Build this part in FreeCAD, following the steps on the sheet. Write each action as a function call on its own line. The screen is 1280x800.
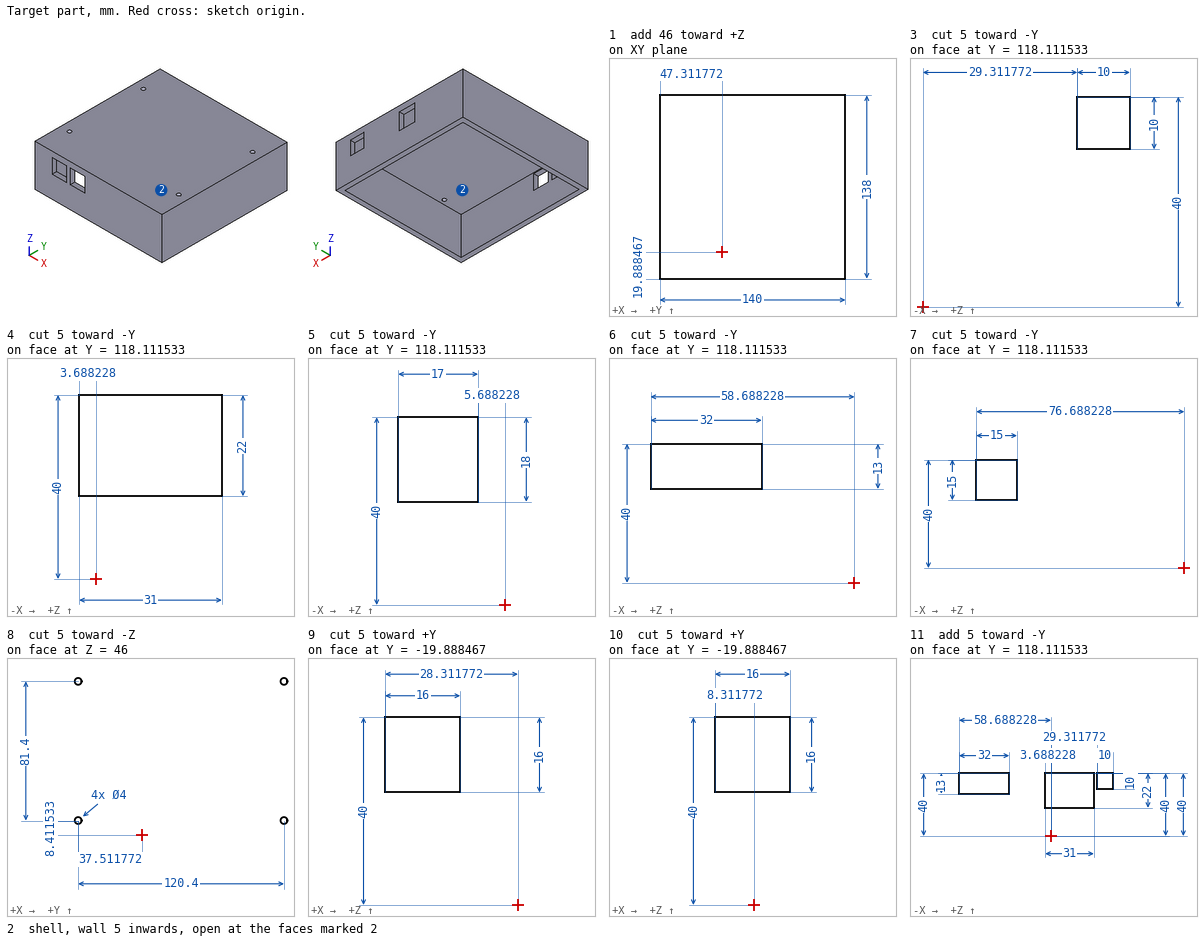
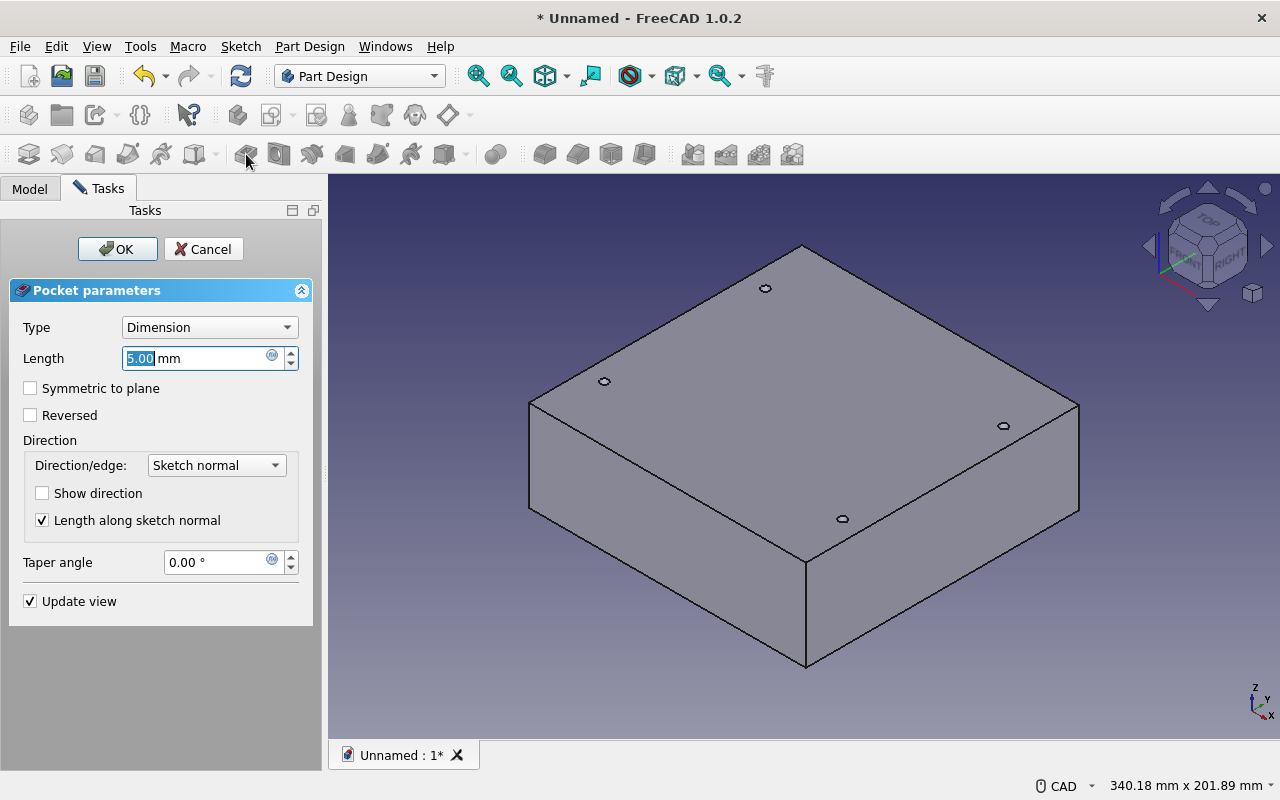
text(5)
key(Tab)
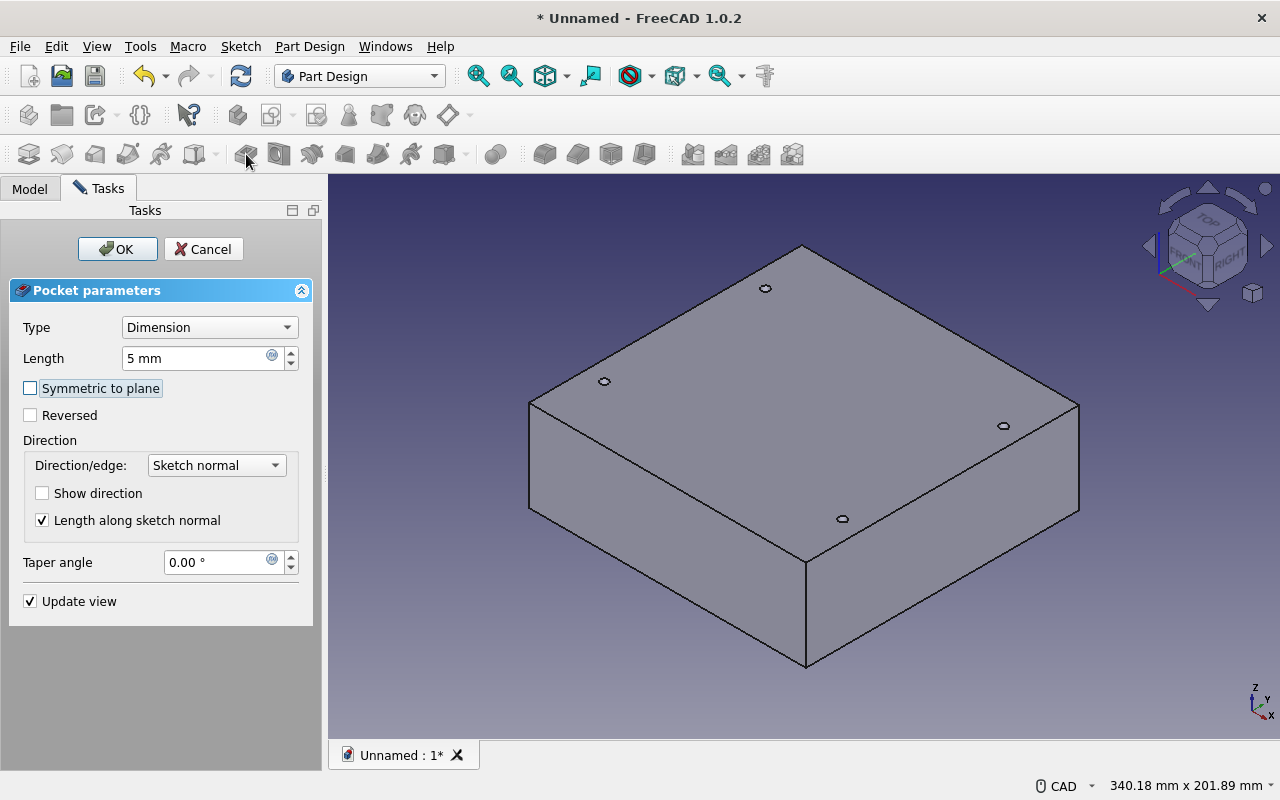
click(118, 249)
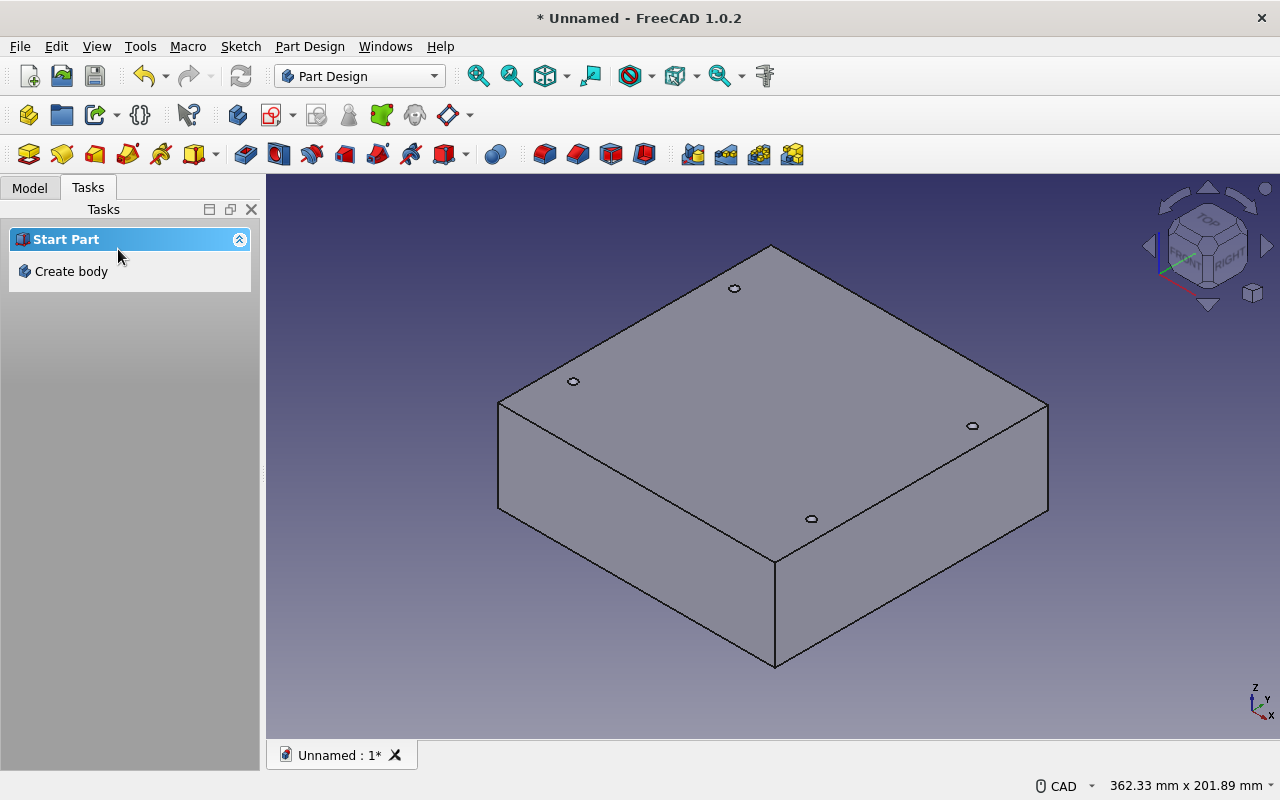
click(716, 580)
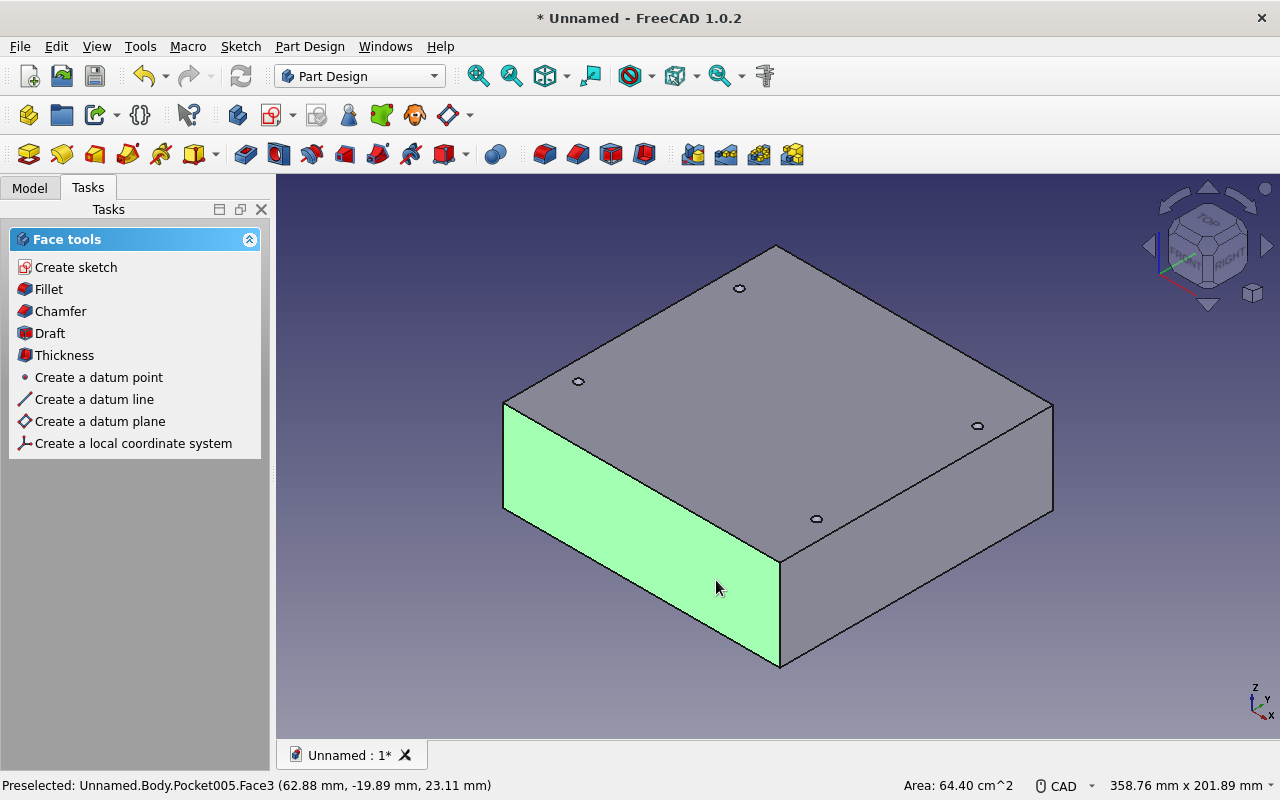
click(270, 116)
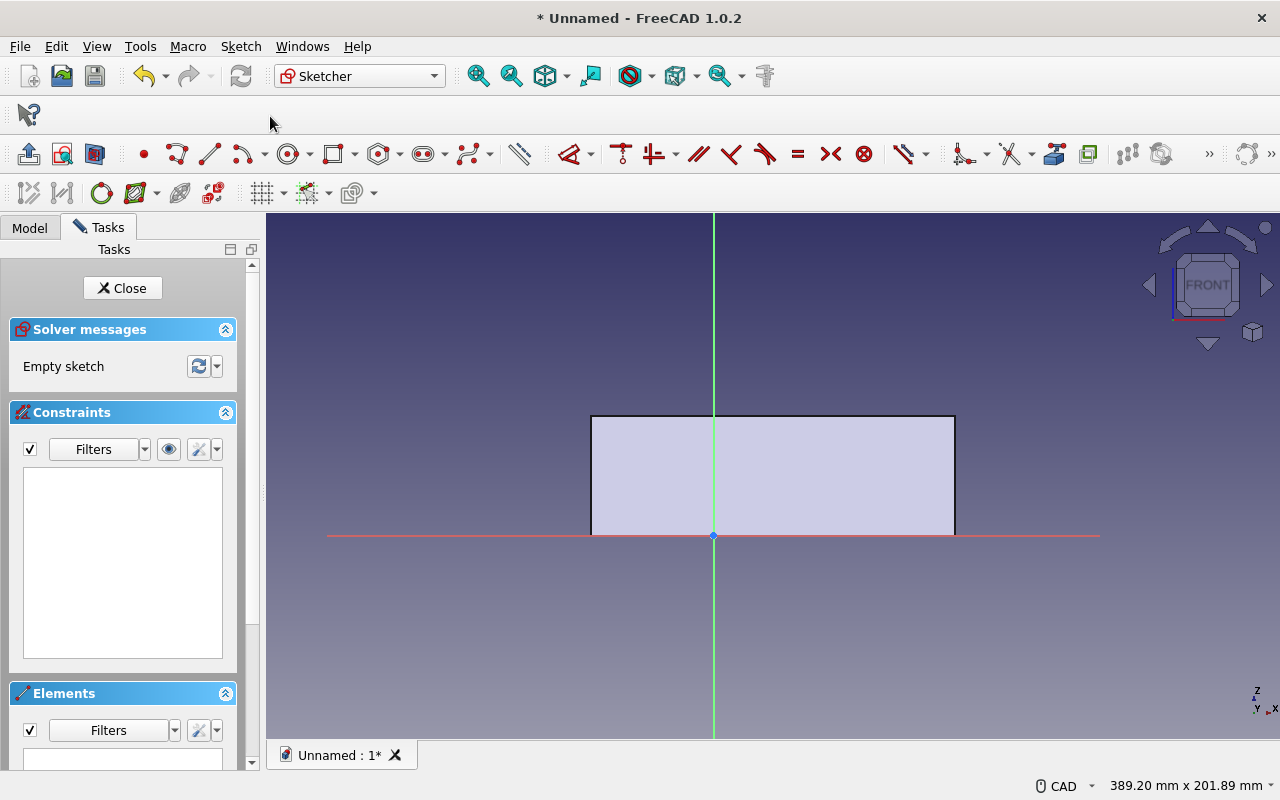
scroll(654, 449, up, 10)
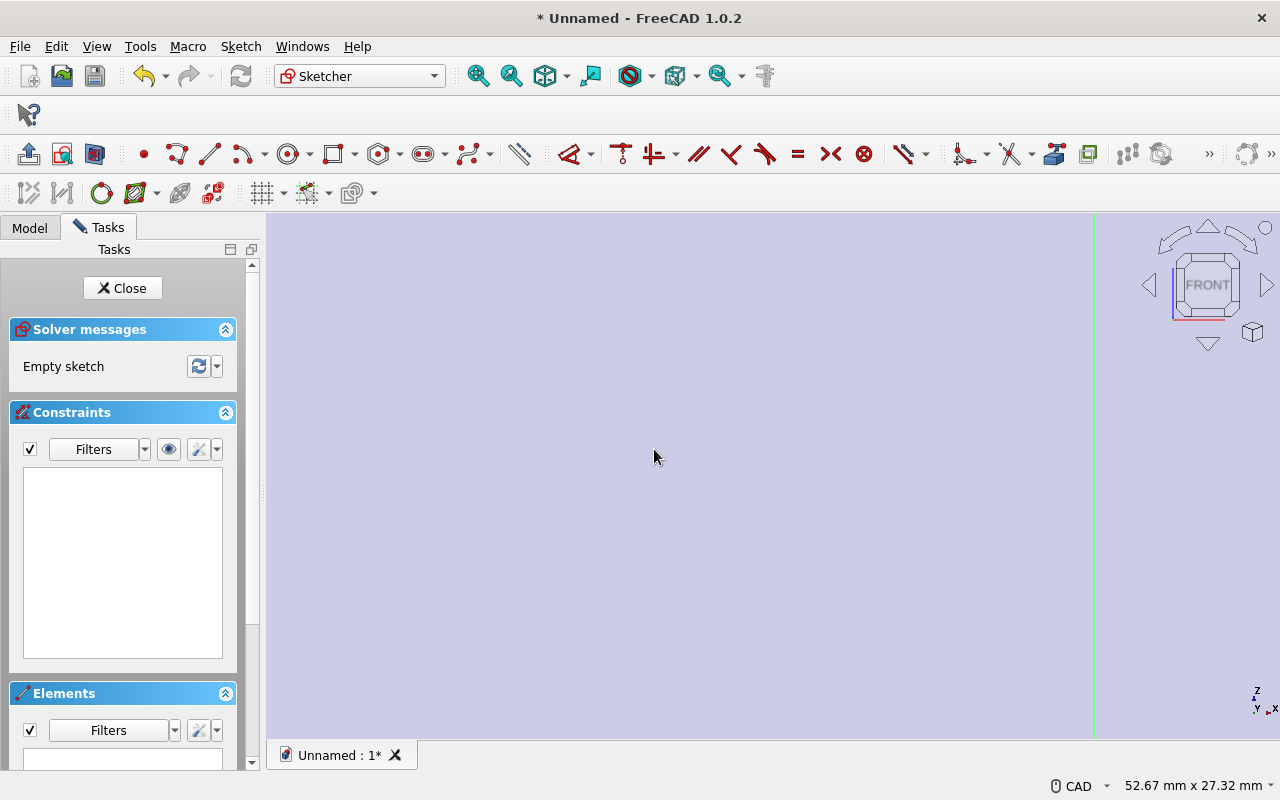
key(g)
key(r)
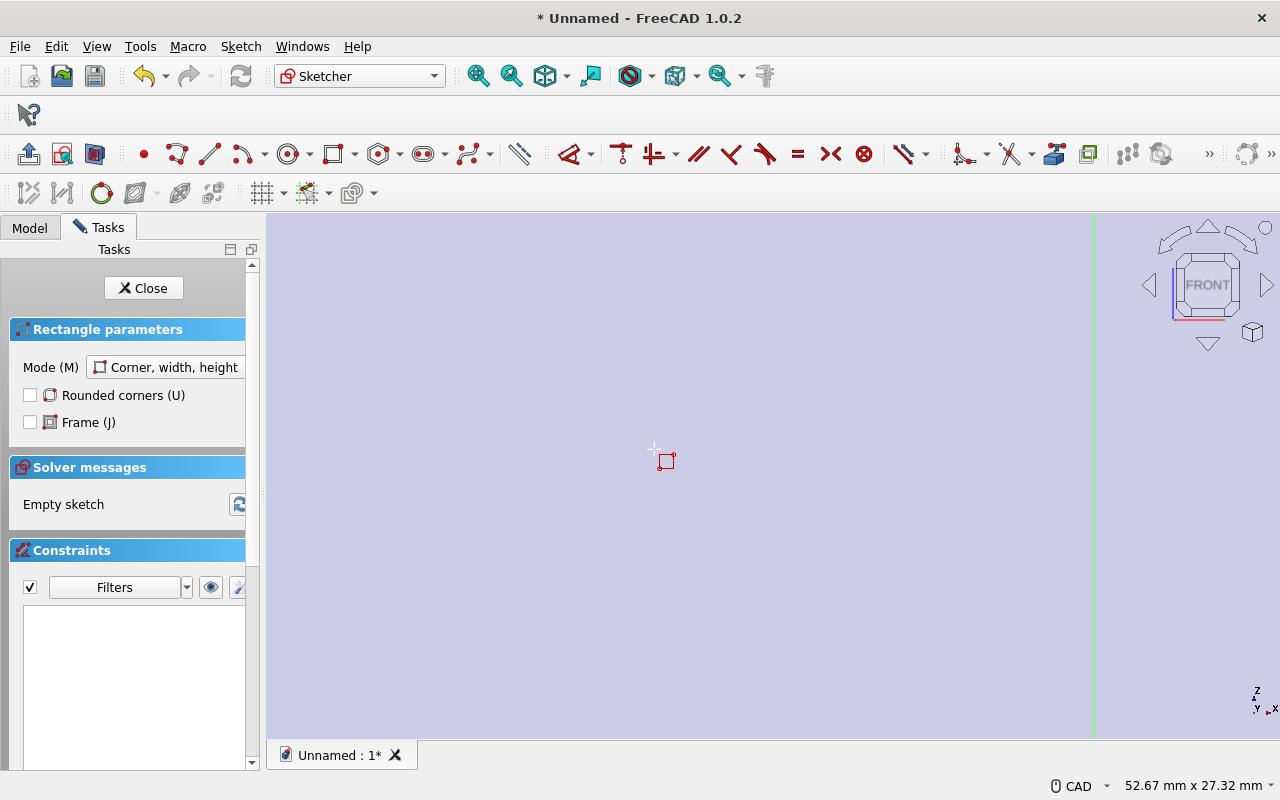
click(549, 318)
move(857, 626)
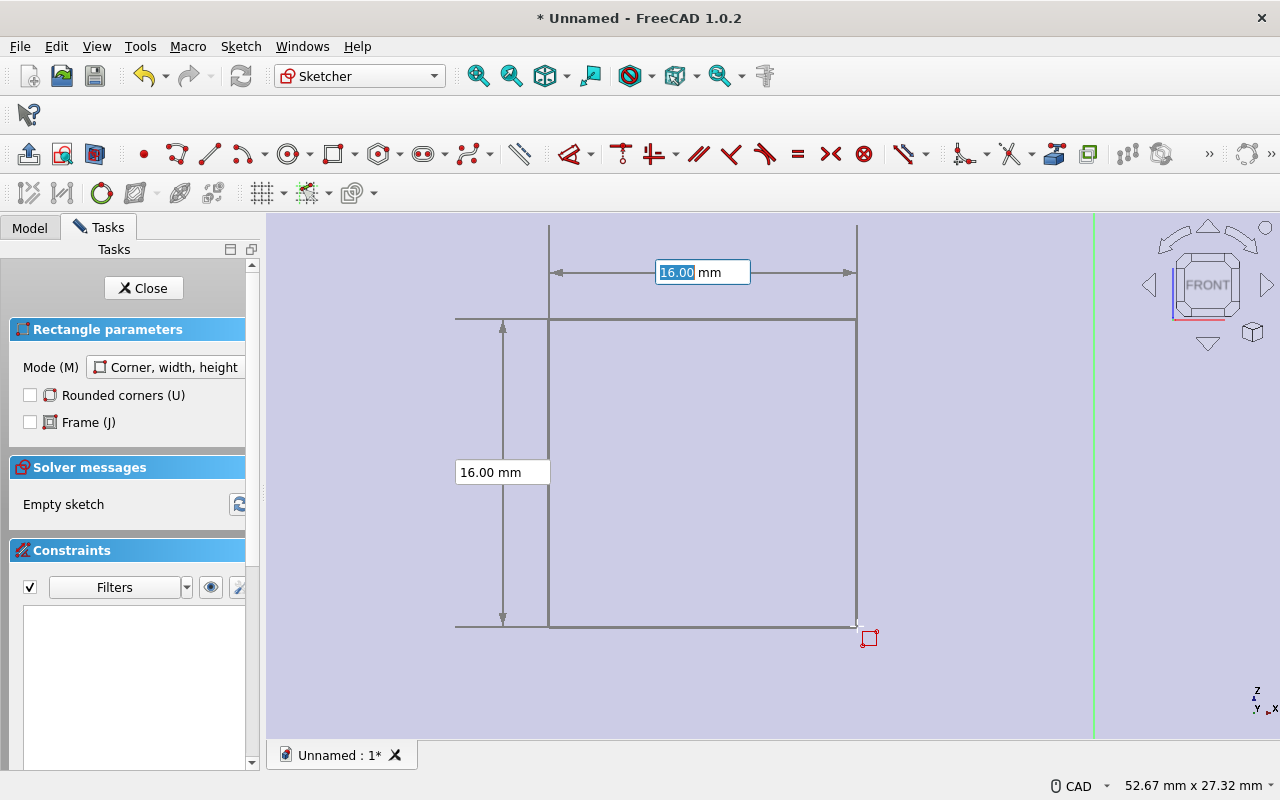
text(16)
key(Tab)
text(16)
key(Return)
key(Escape)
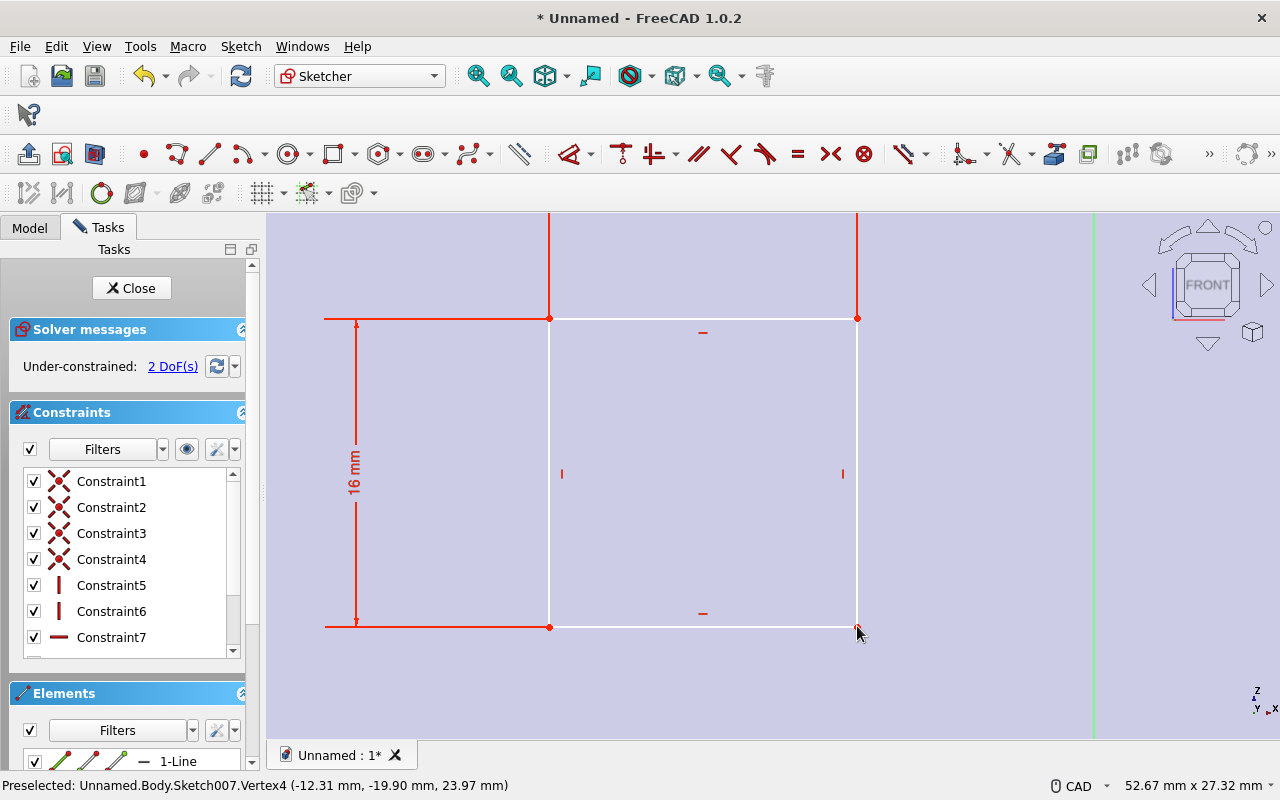
click(568, 154)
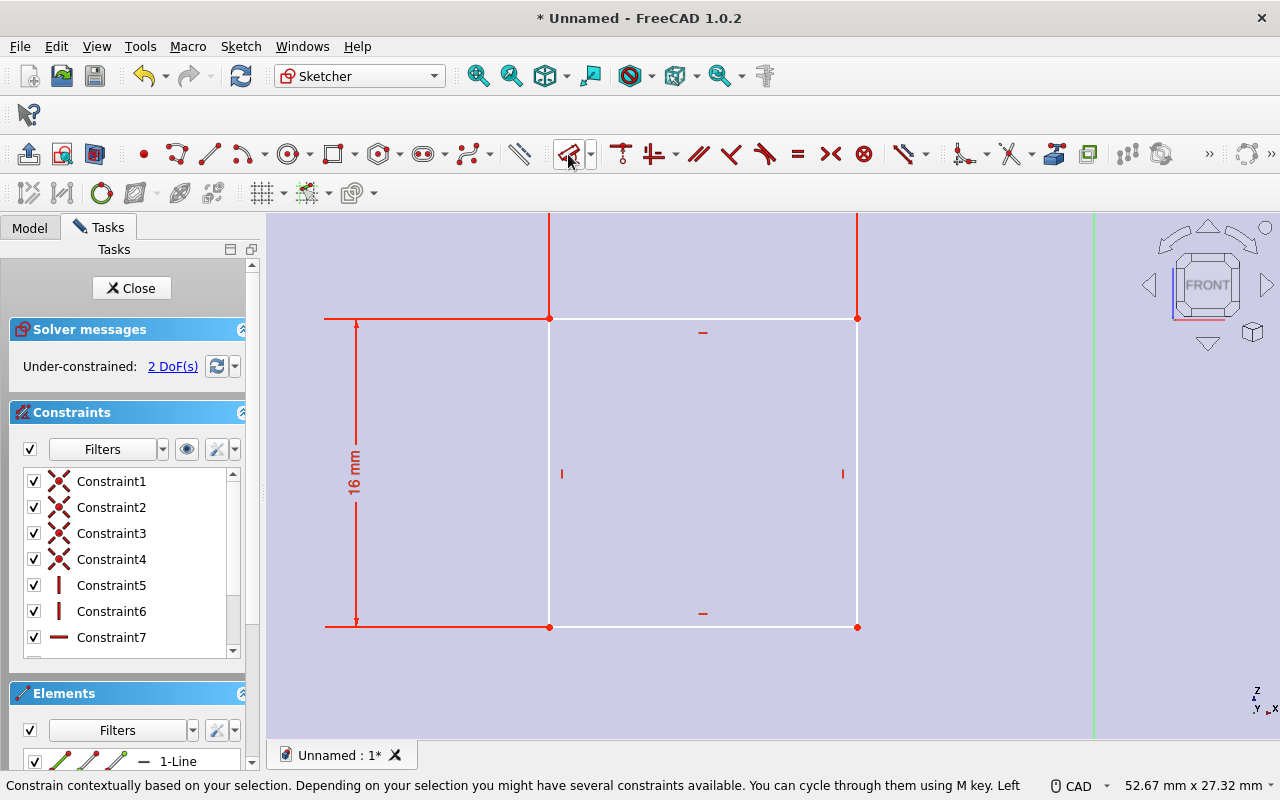
click(549, 319)
click(515, 515)